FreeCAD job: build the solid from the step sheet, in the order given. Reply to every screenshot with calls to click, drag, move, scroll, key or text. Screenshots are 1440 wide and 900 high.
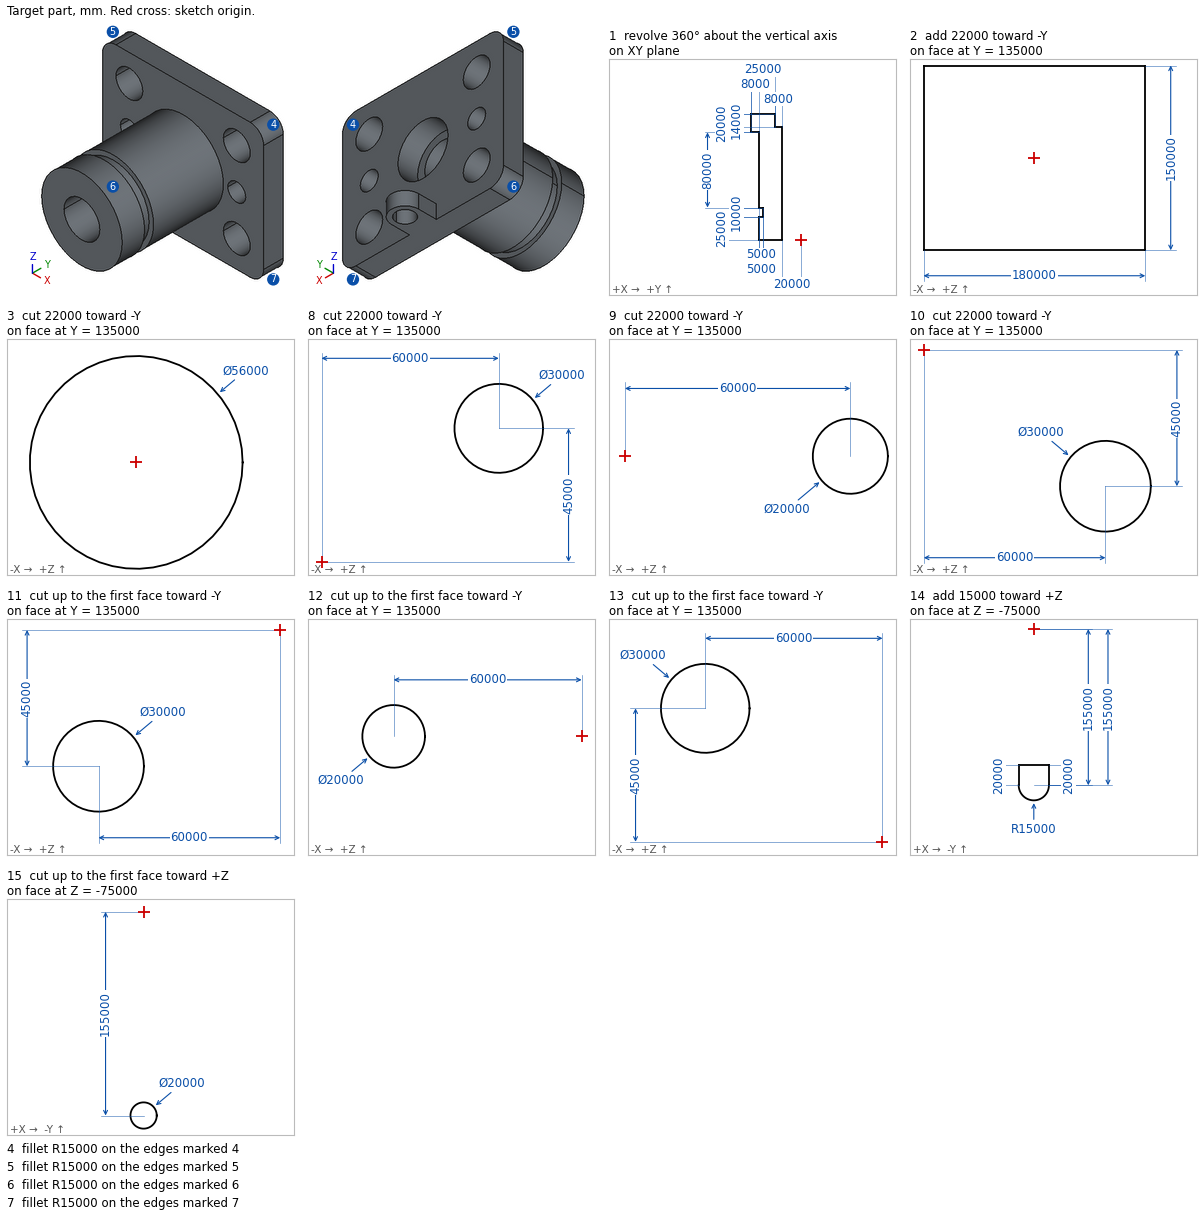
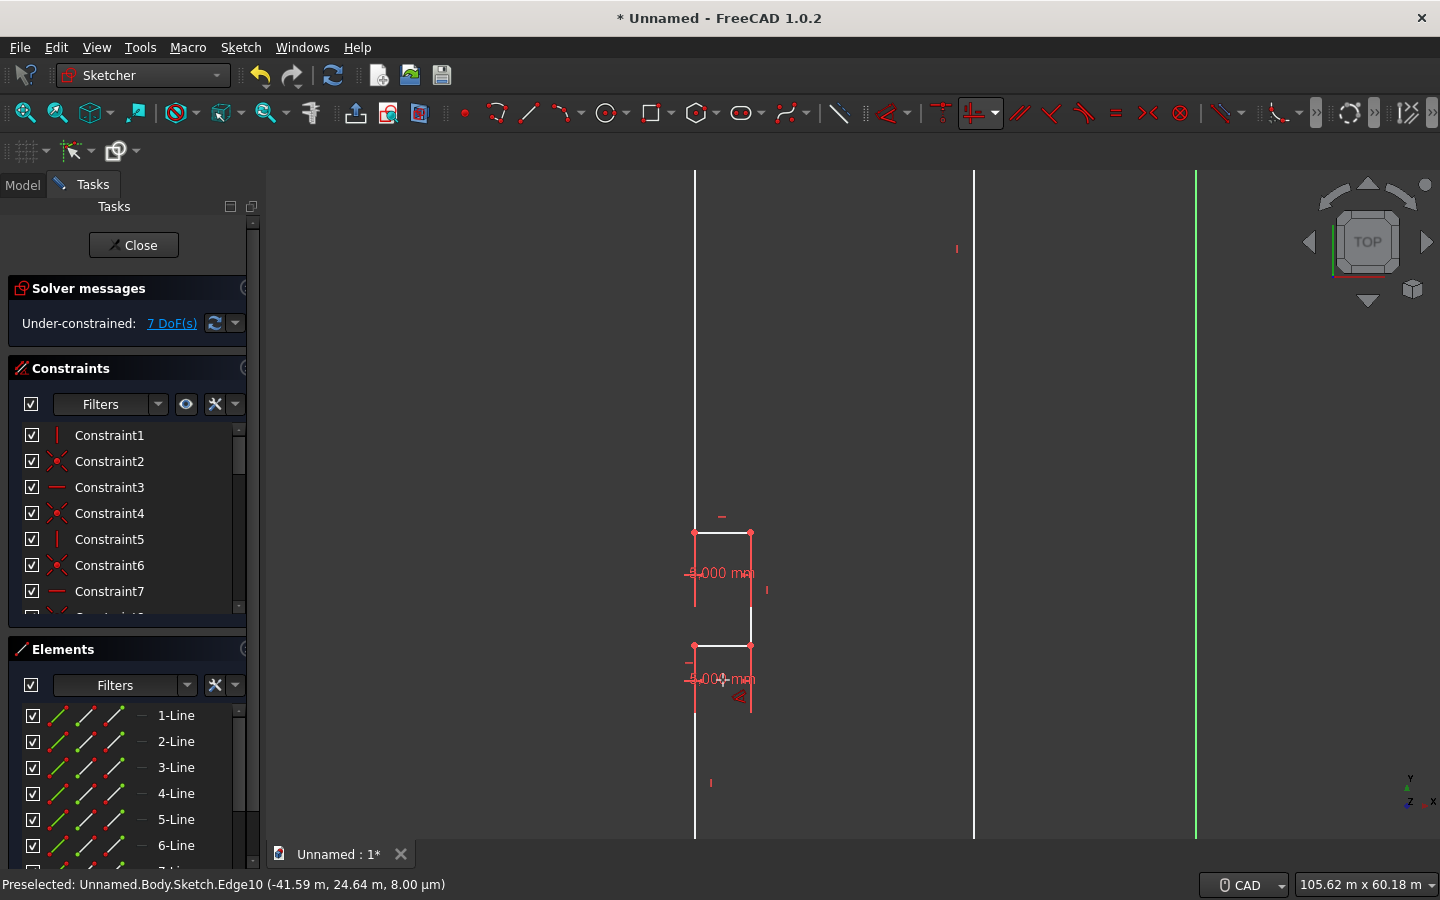
scroll(734, 649, down, 6)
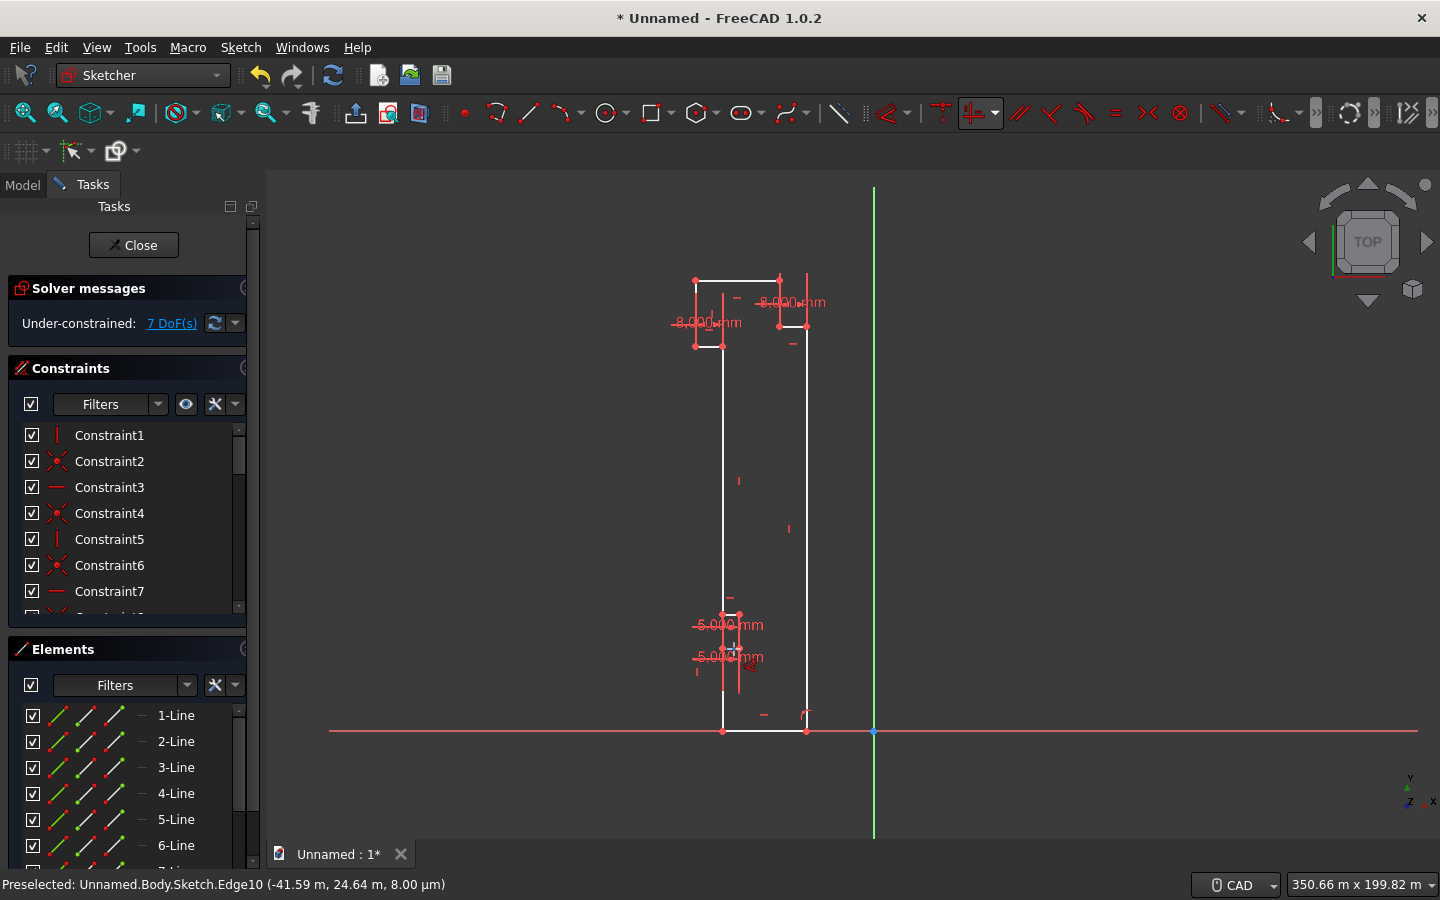
click(780, 313)
click(722, 304)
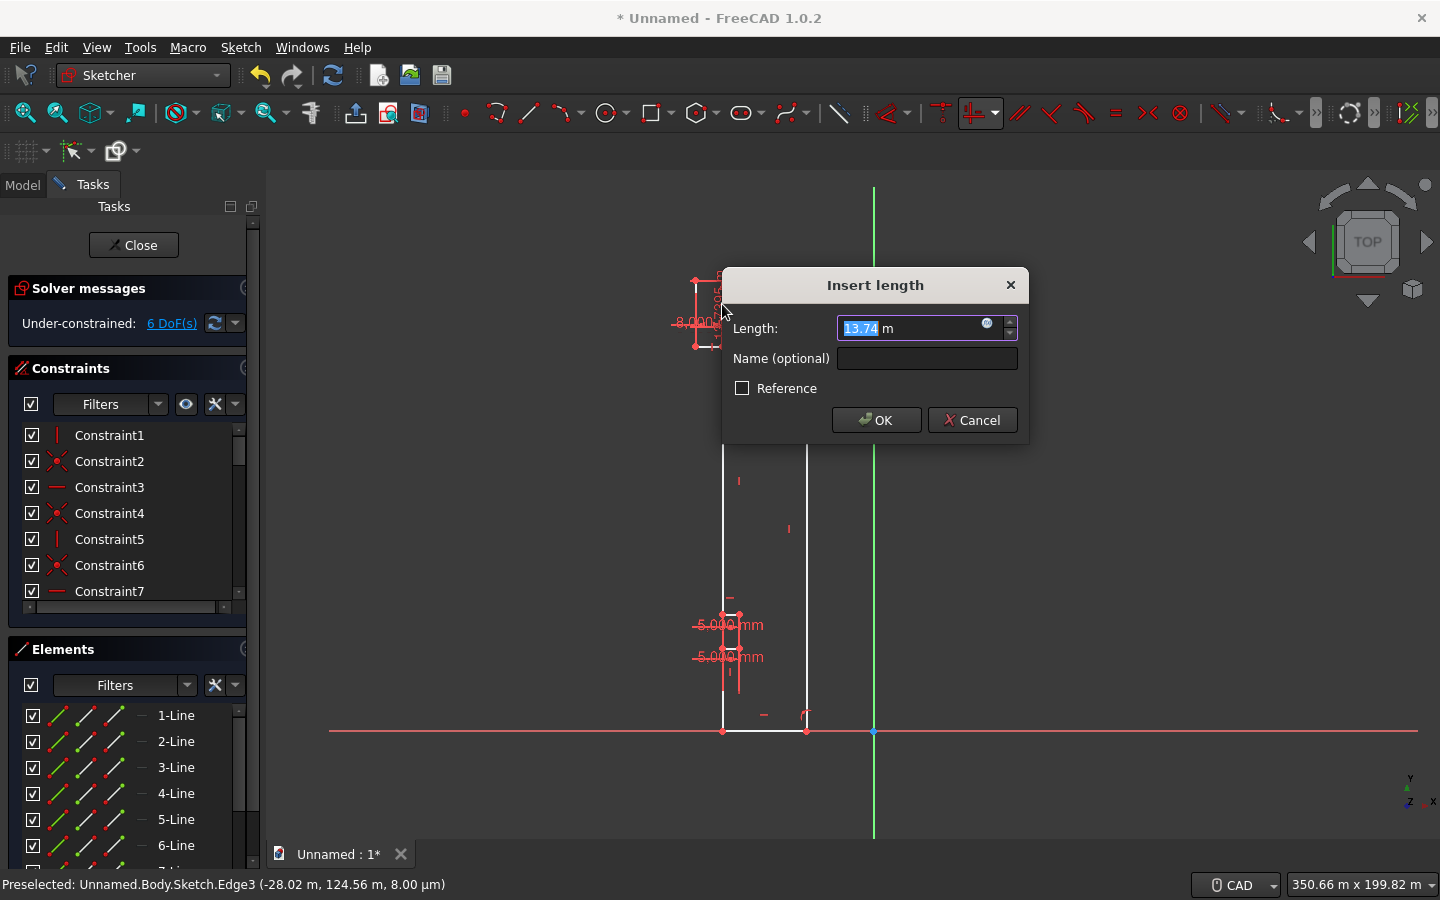
key(ctrl+a)
text(14000 mm)
key(Return)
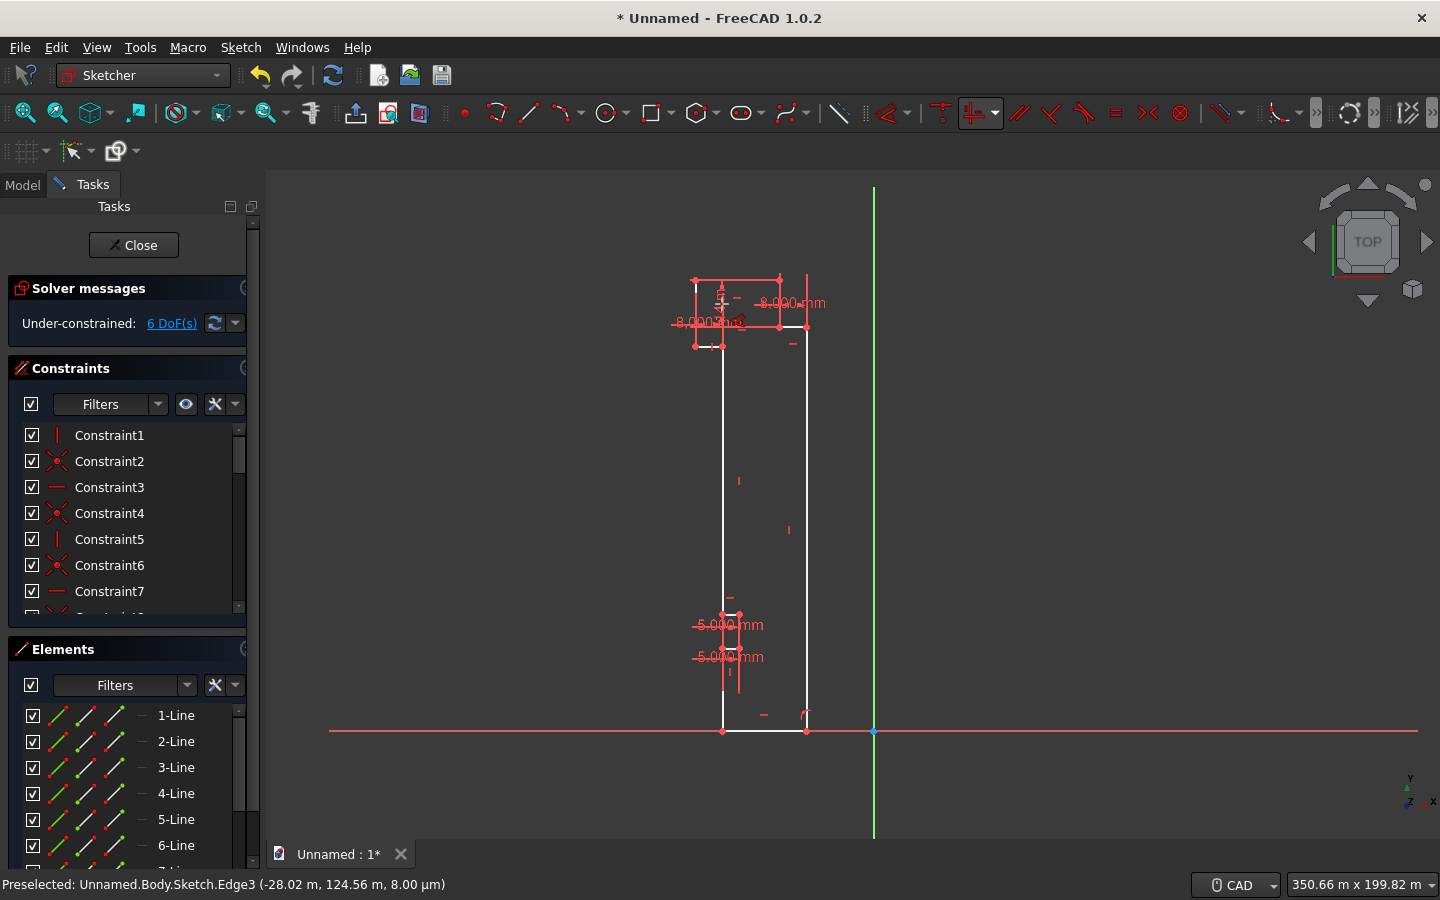
click(755, 280)
click(738, 246)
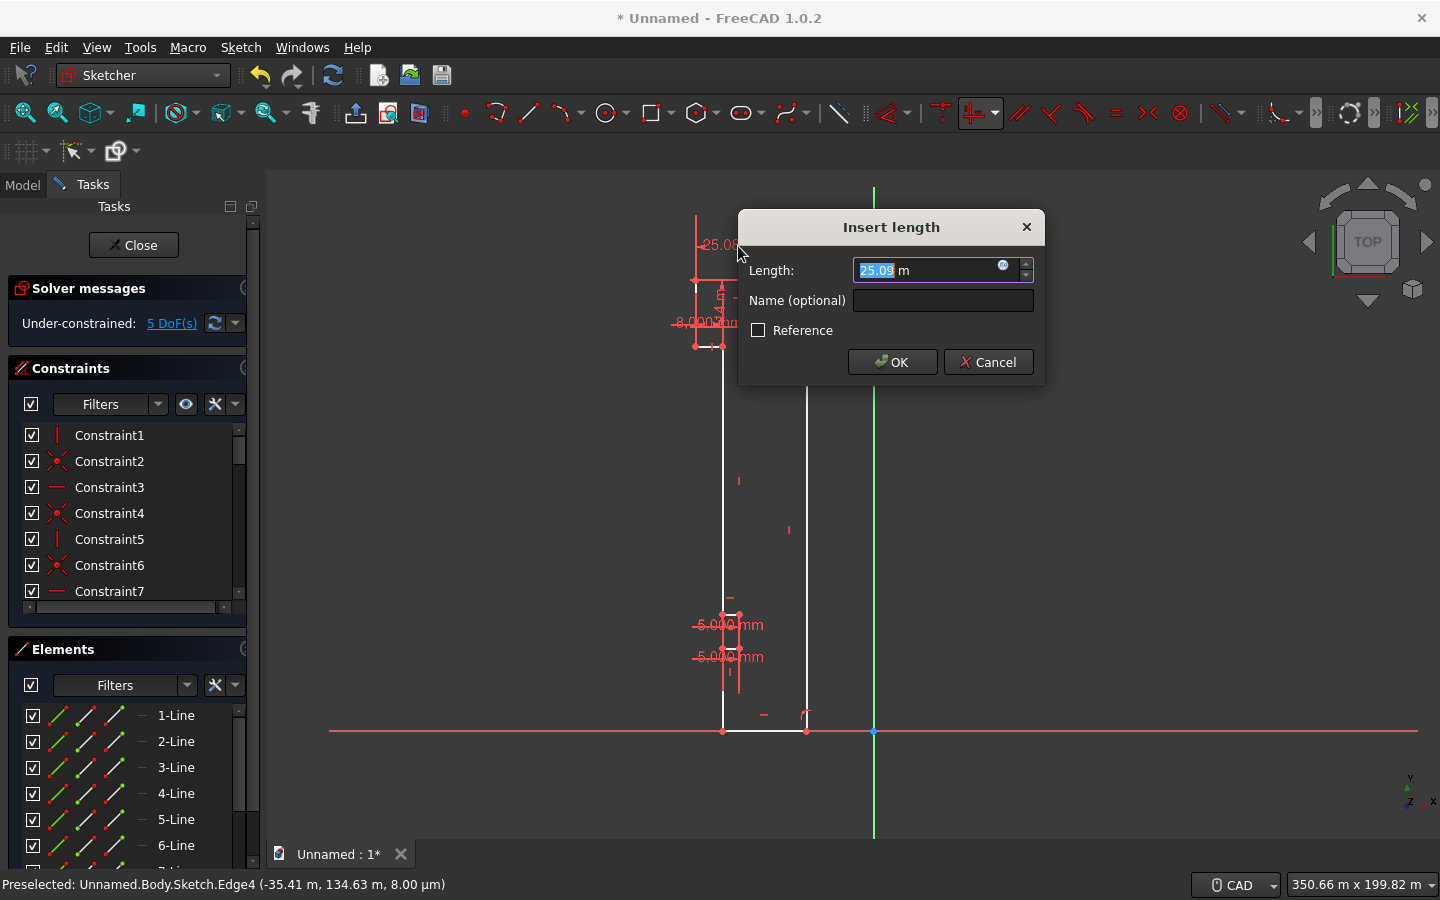
key(ctrl+a)
text(25000 mm)
key(Return)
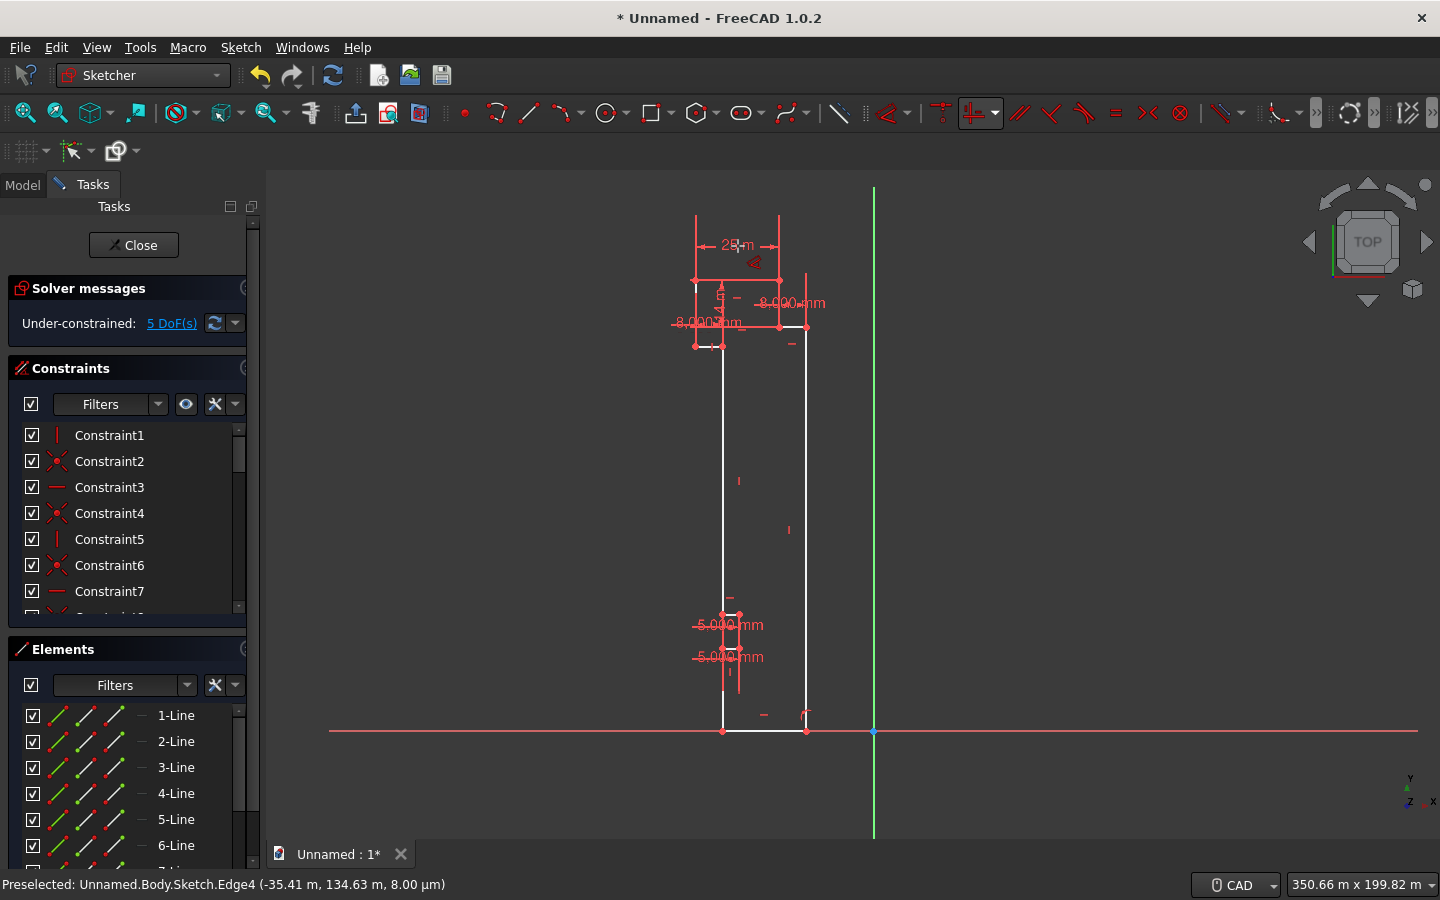
click(696, 300)
click(638, 313)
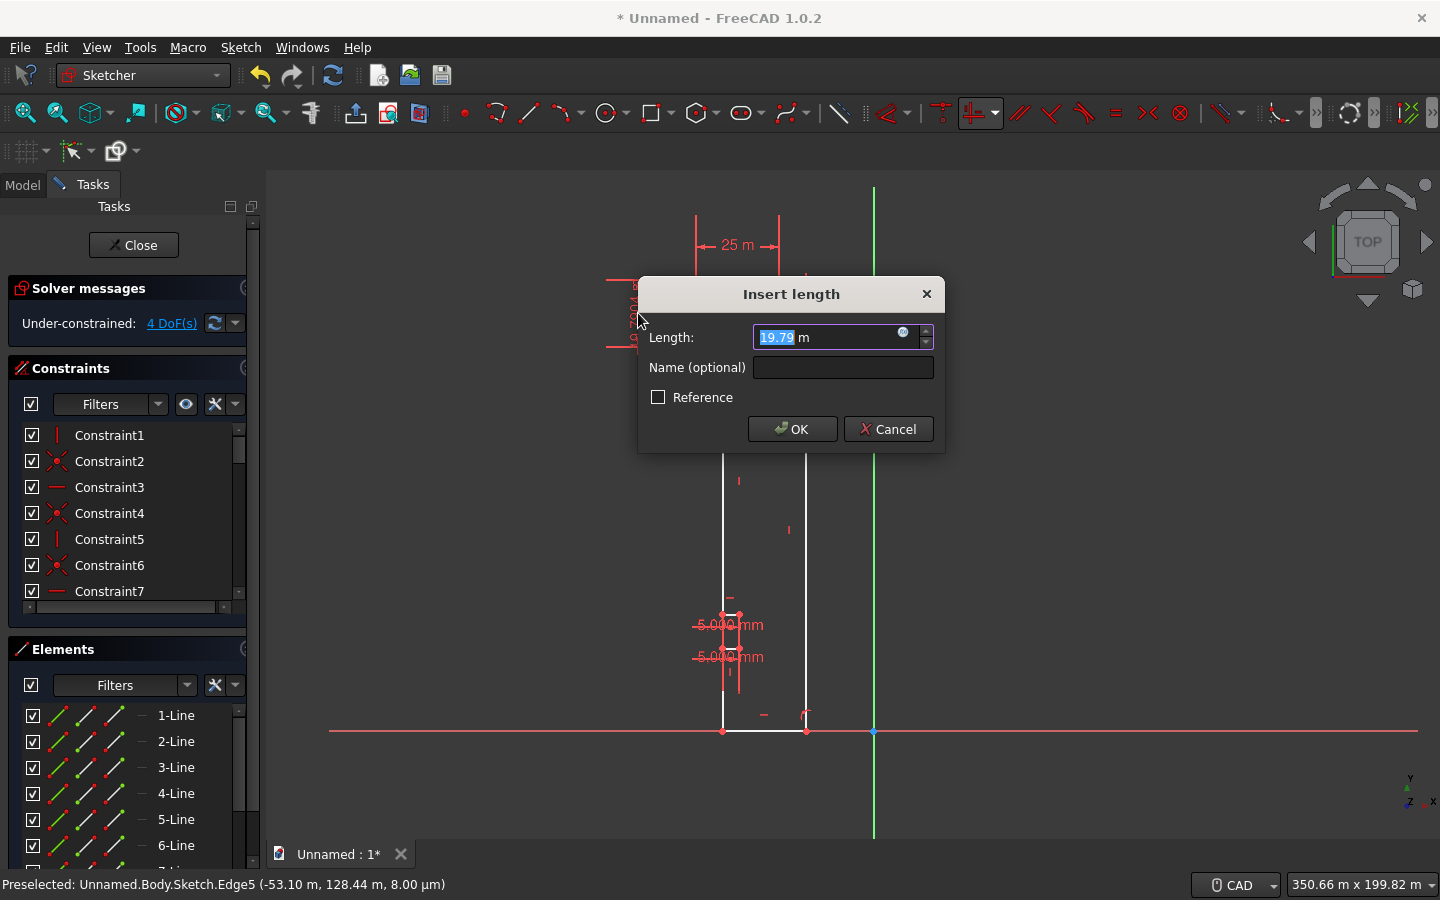
key(ctrl+a)
text(20000 mm)
key(Return)